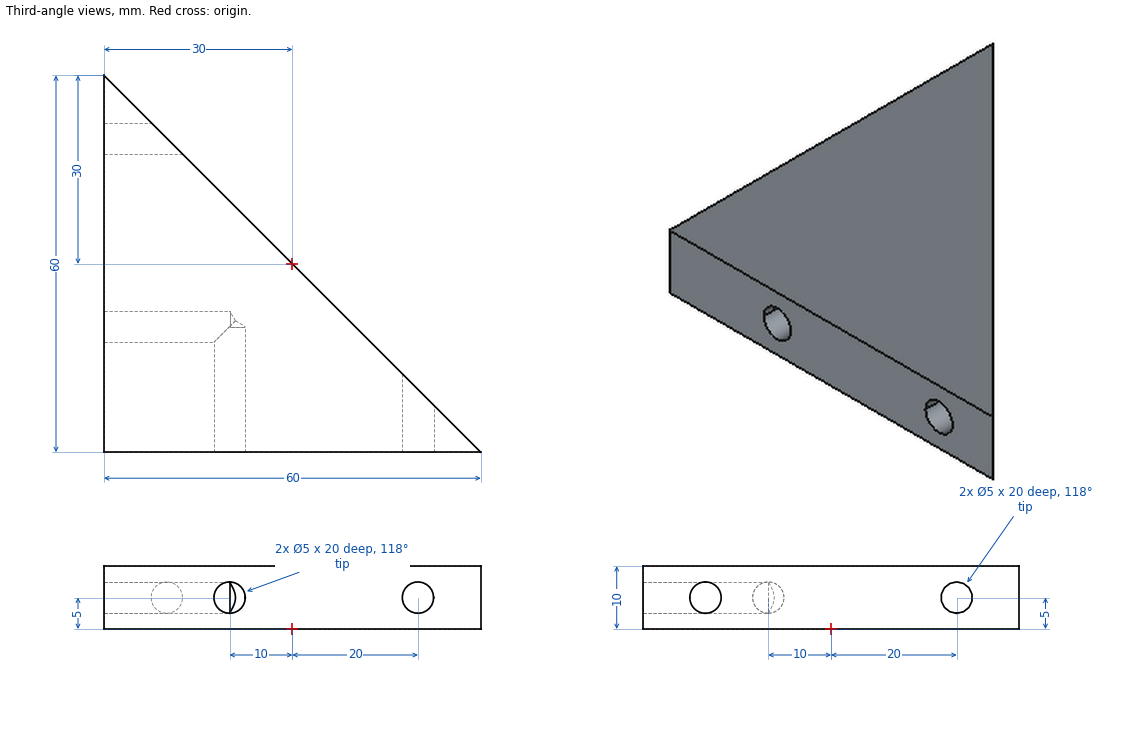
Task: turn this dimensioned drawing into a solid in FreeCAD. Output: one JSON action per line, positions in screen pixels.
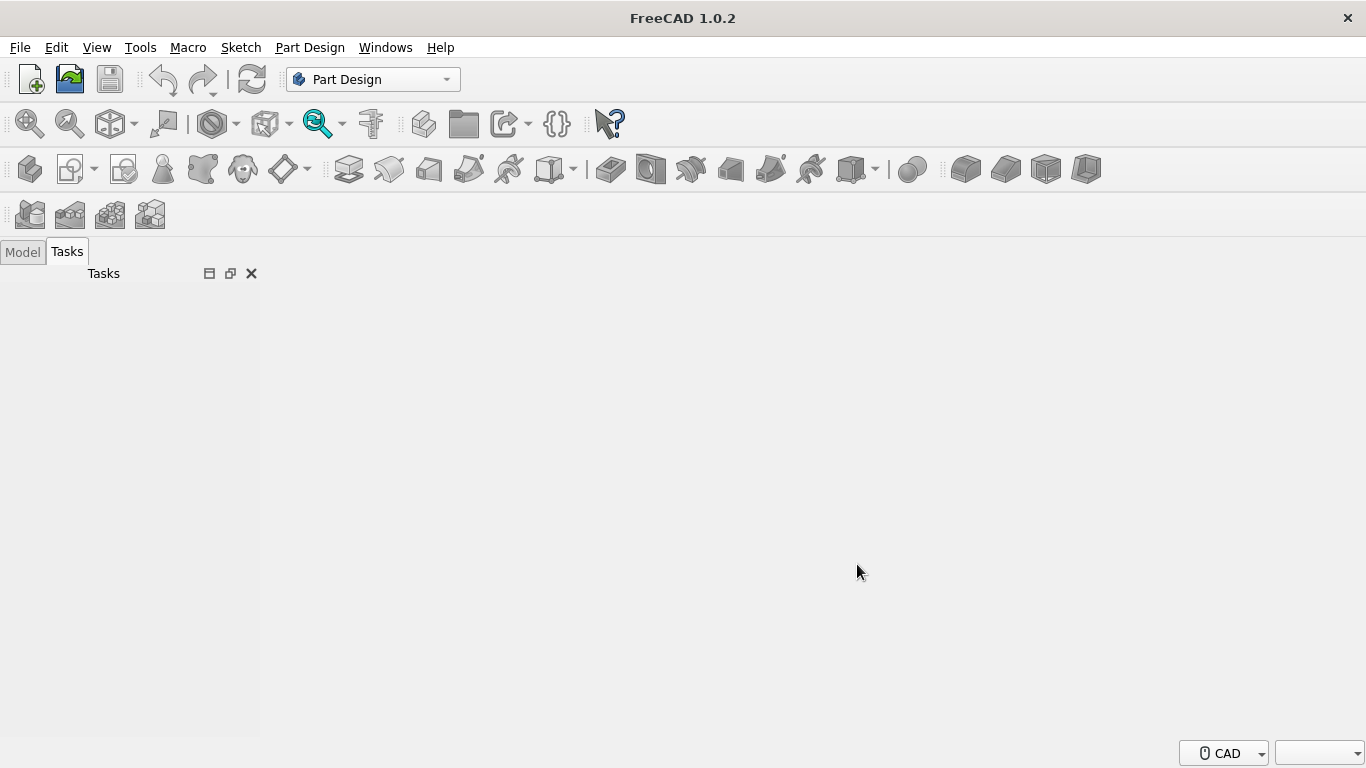
{"action": "key", "text": "ctrl+n"}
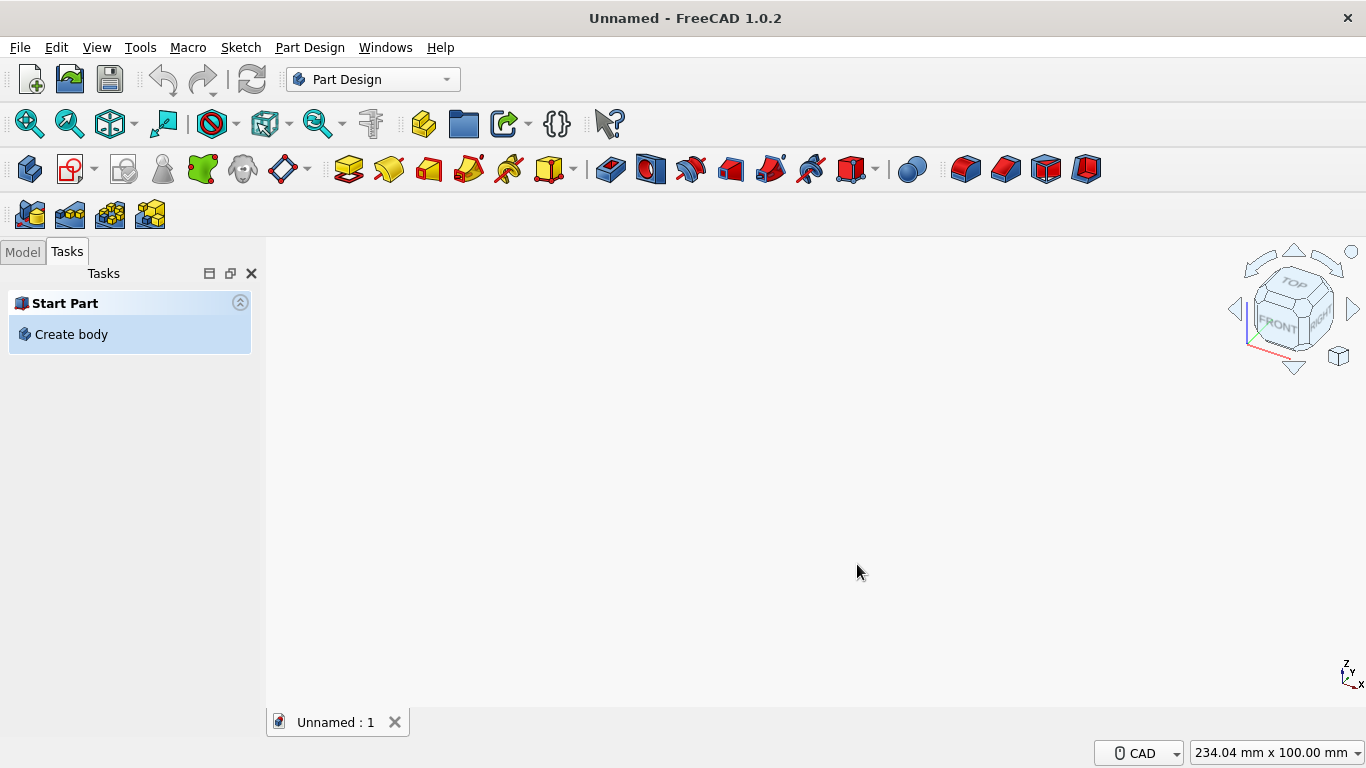
{"action": "left_click", "coordinate": [70, 170]}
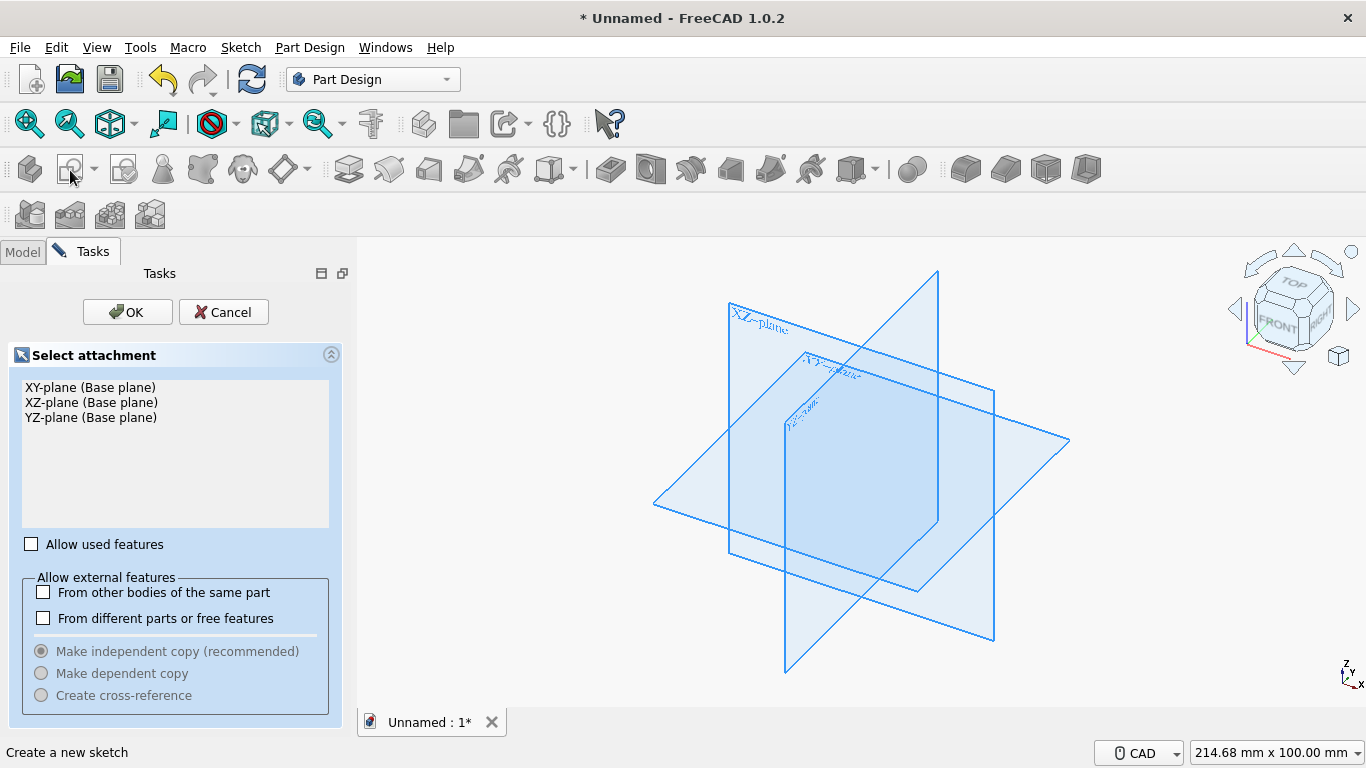
{"action": "left_click", "coordinate": [82, 388]}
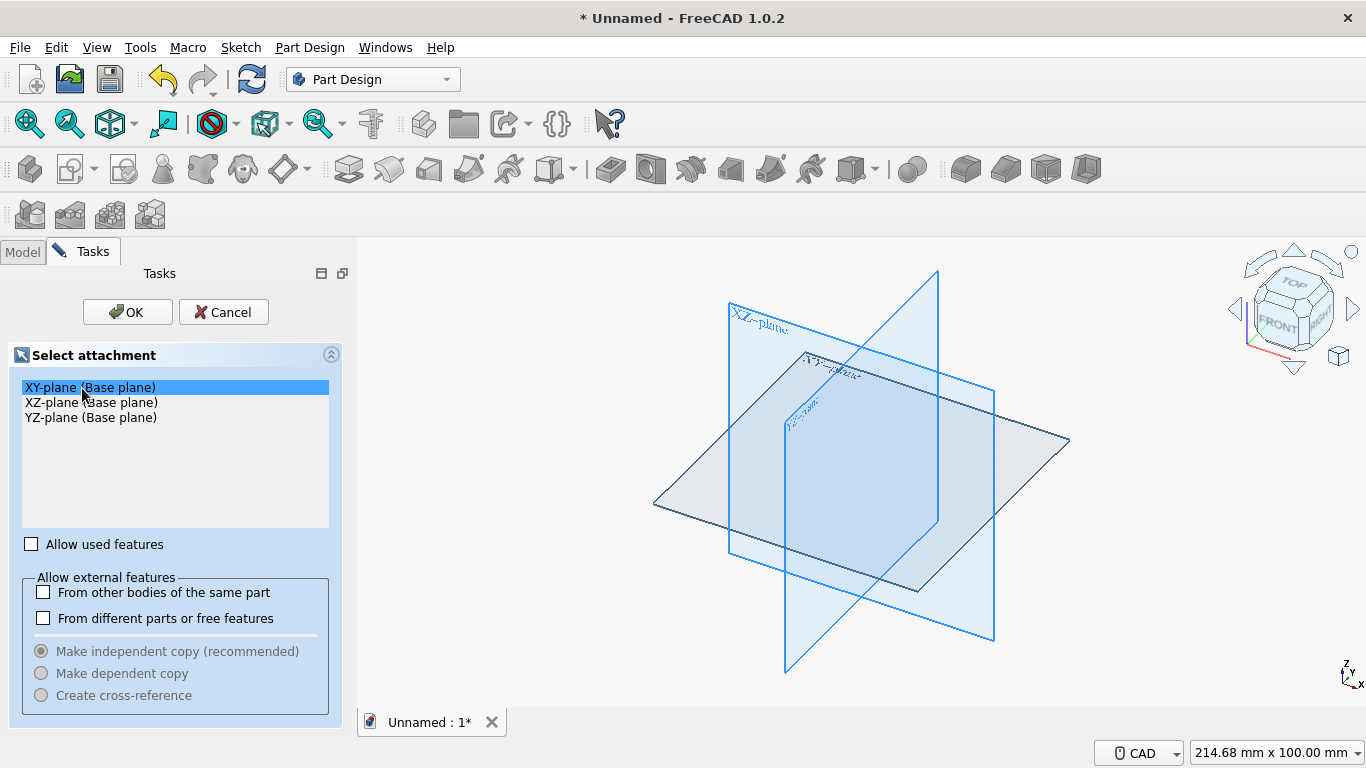
{"action": "left_click", "coordinate": [128, 312]}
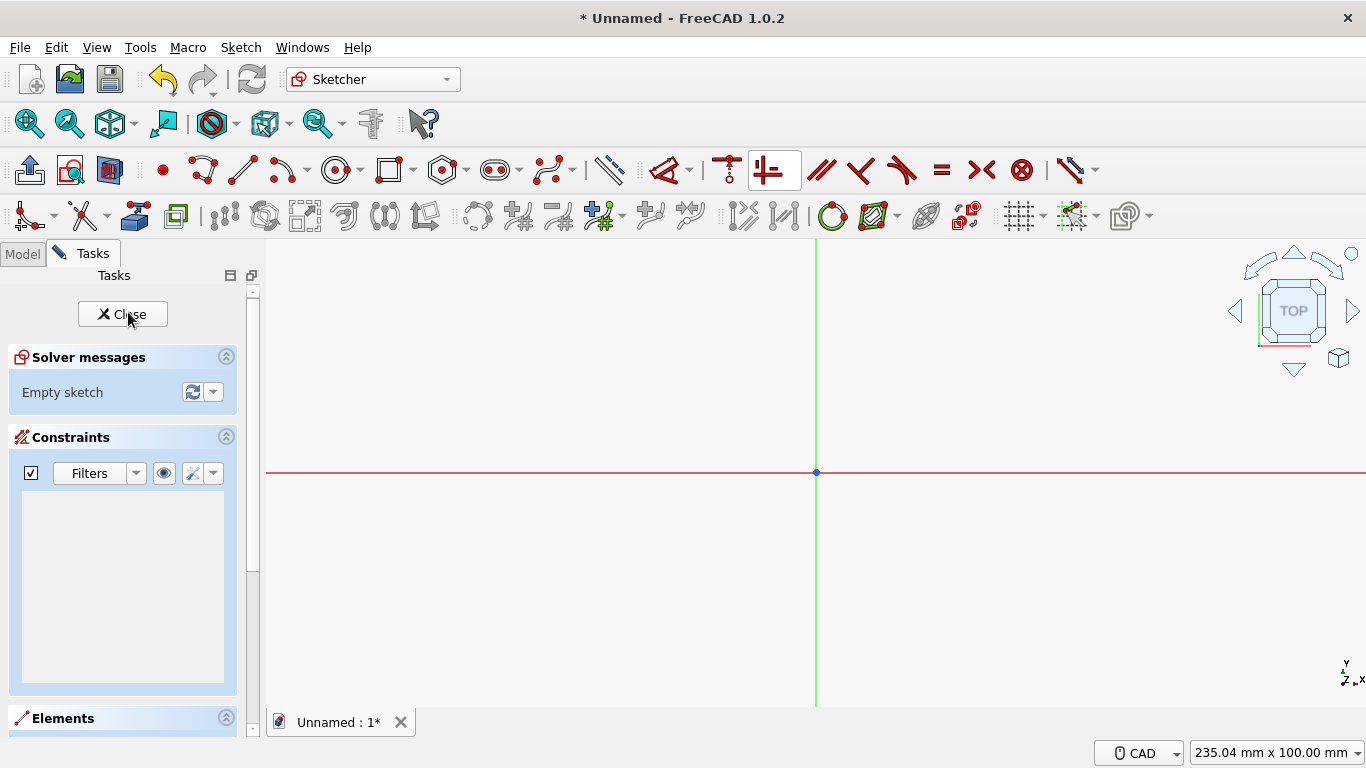
{"action": "key", "text": "g m"}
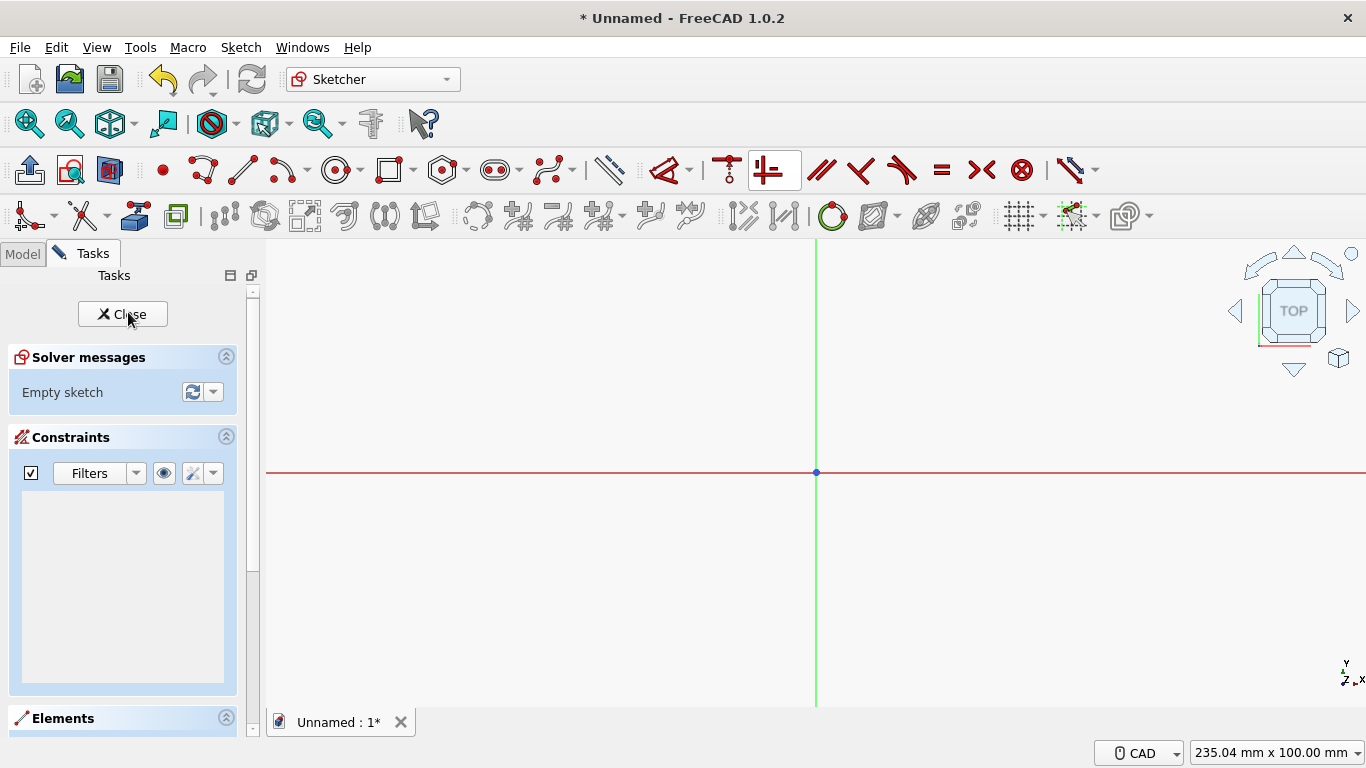
{"action": "left_click", "coordinate": [676, 333]}
{"action": "left_click", "coordinate": [676, 613]}
{"action": "left_click", "coordinate": [956, 613]}
{"action": "left_click", "coordinate": [676, 334]}
{"action": "key", "text": "Escape"}
{"action": "key", "text": "Escape"}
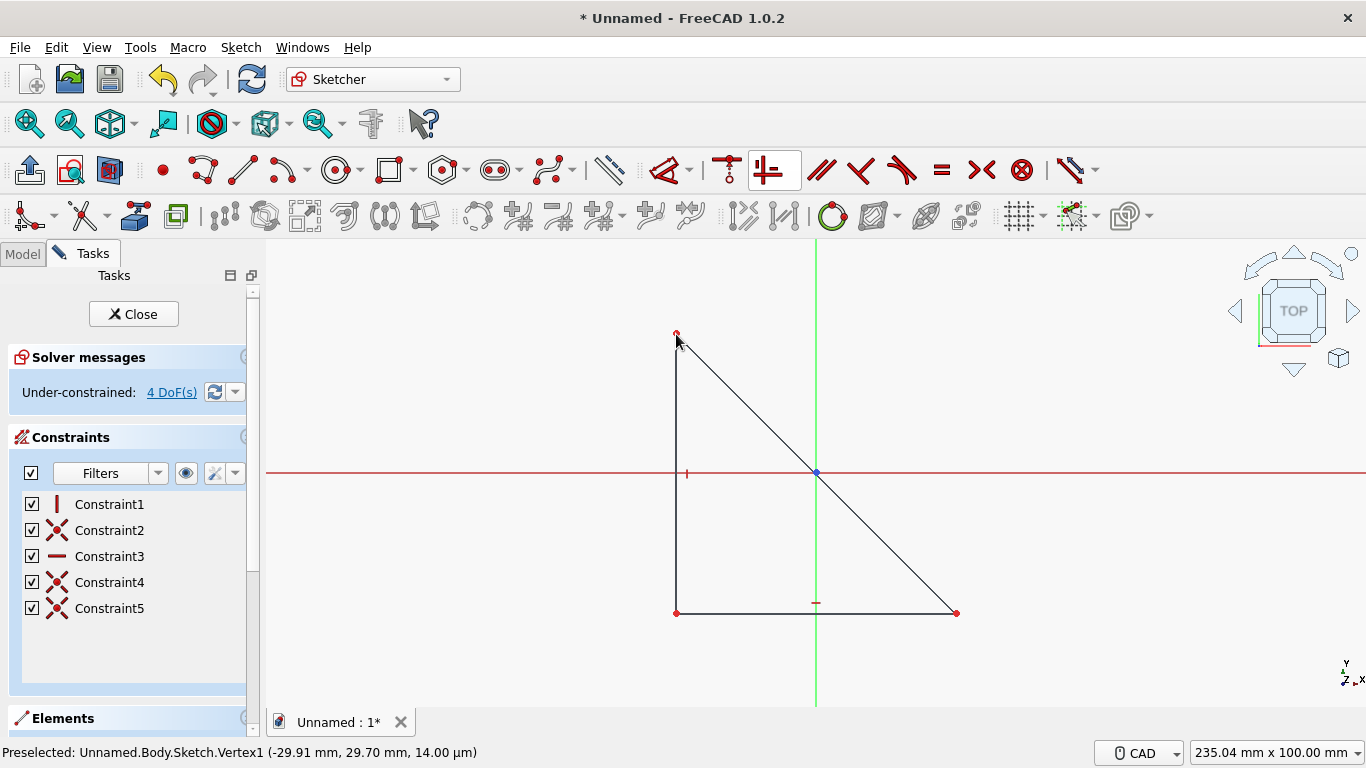
{"action": "left_click", "coordinate": [676, 418]}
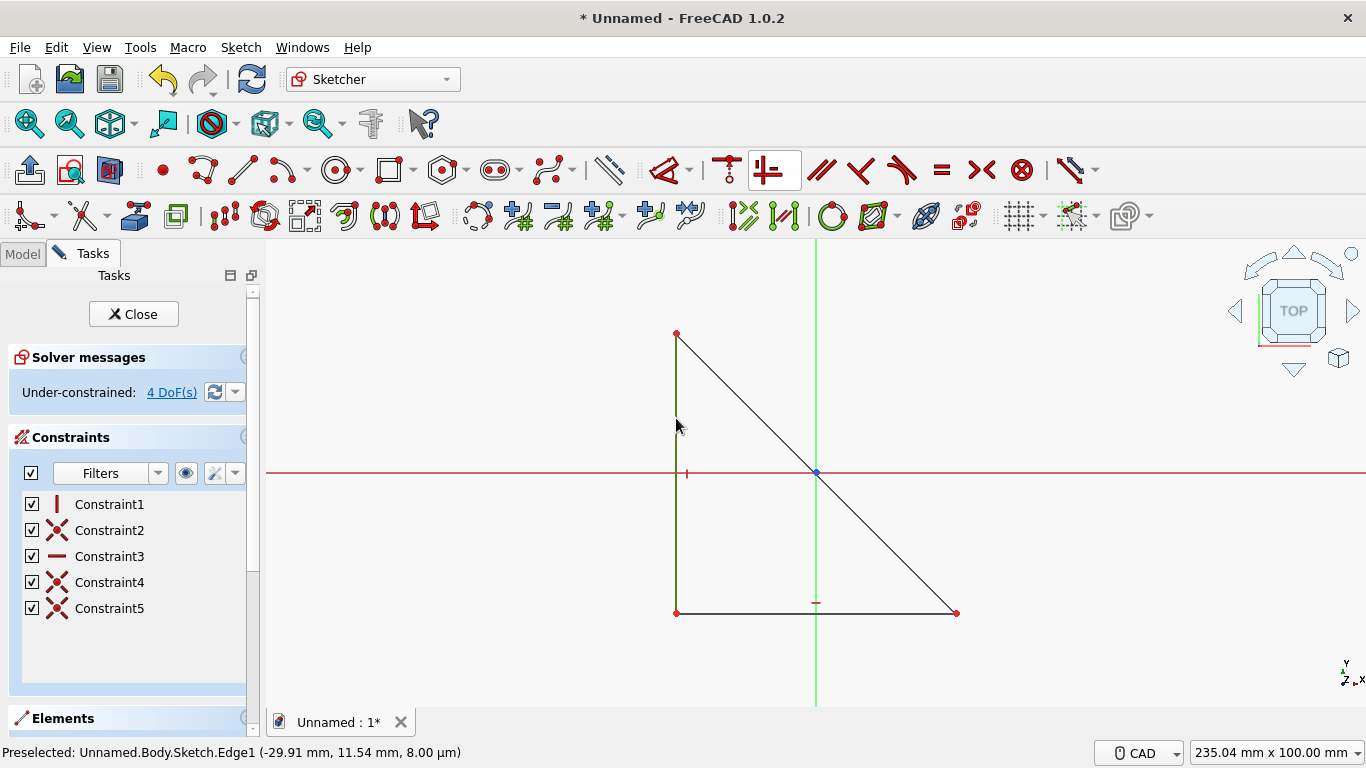
{"action": "left_click", "coordinate": [692, 170]}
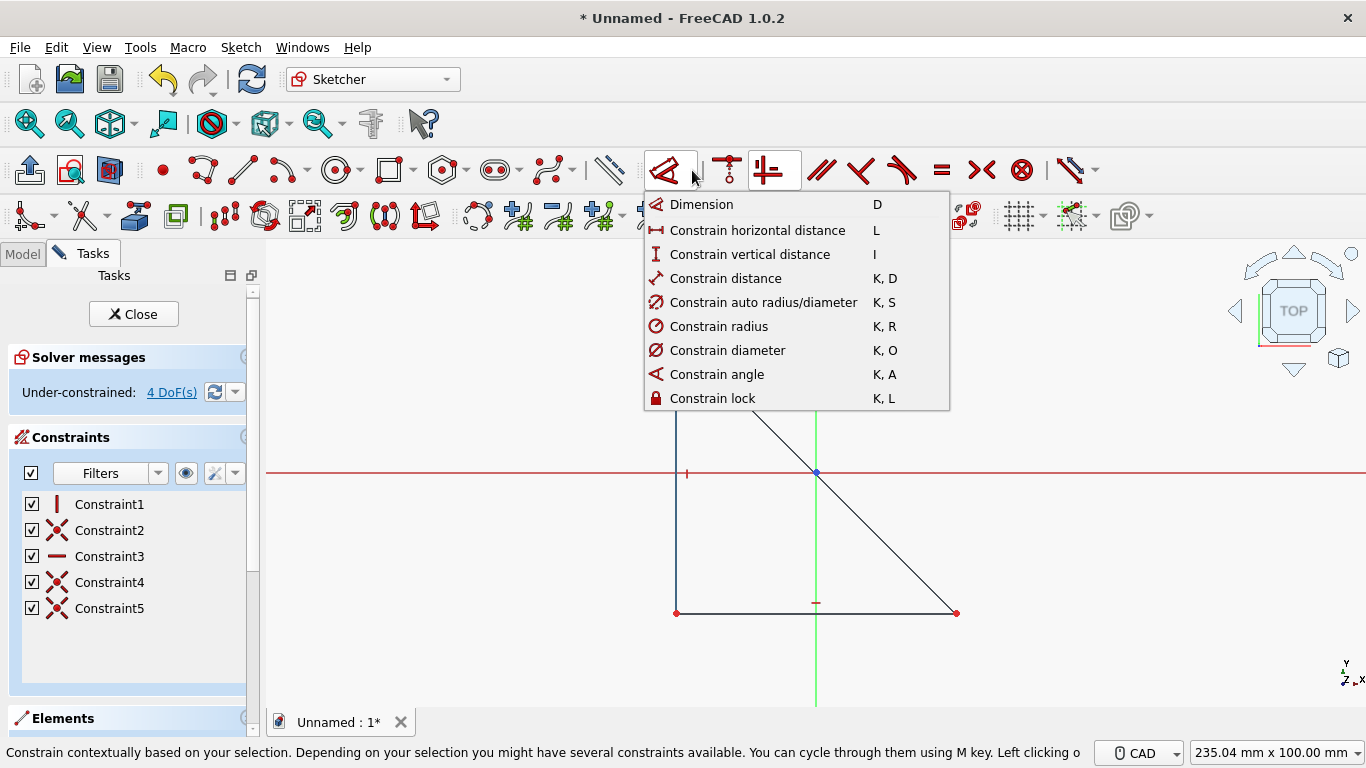
{"action": "left_click", "coordinate": [797, 254]}